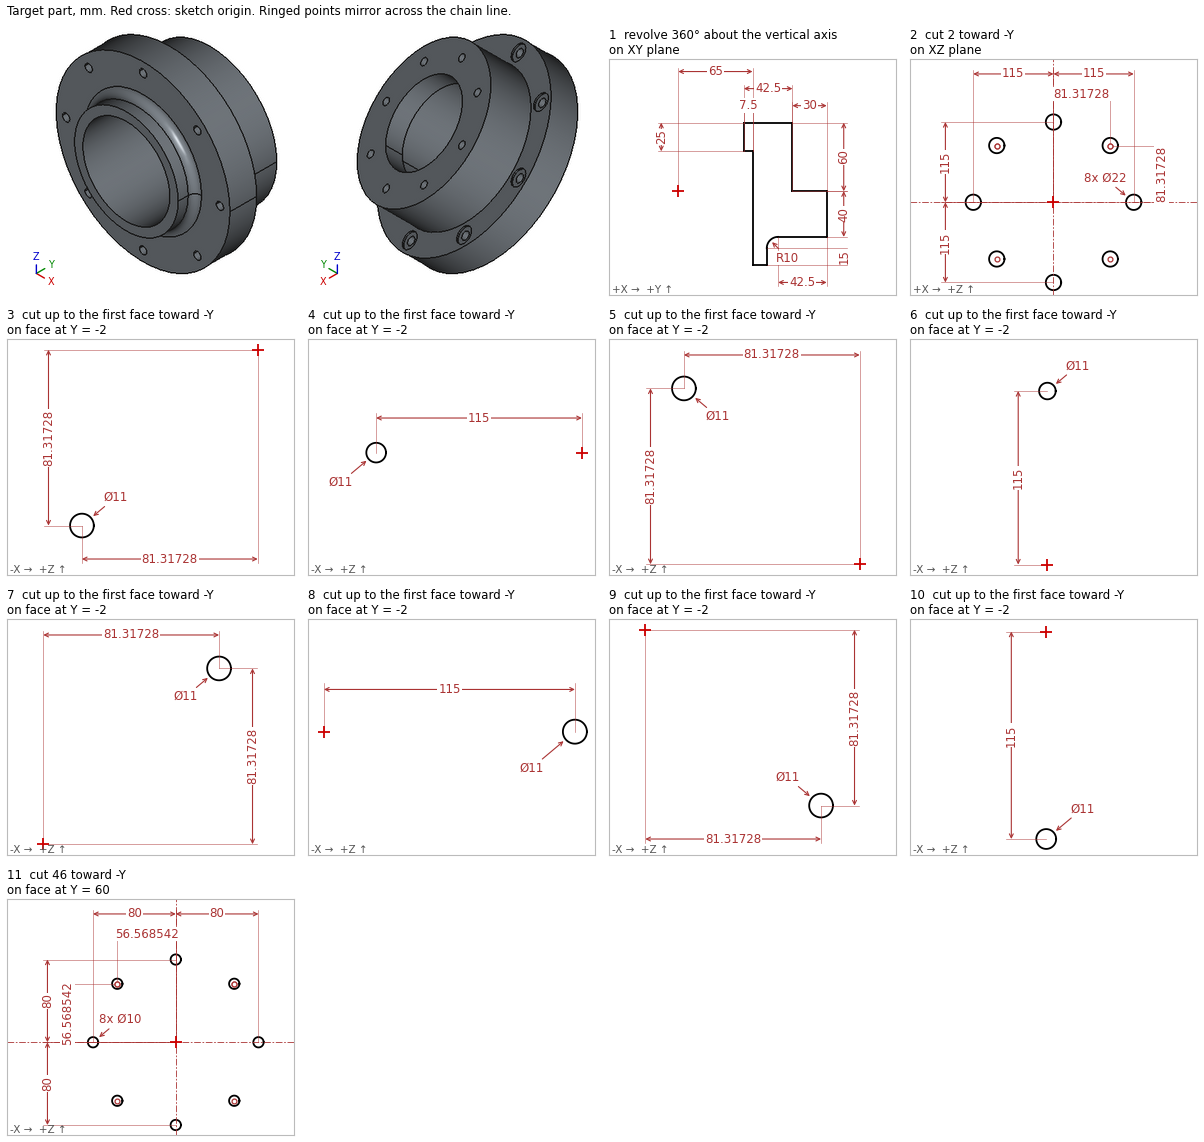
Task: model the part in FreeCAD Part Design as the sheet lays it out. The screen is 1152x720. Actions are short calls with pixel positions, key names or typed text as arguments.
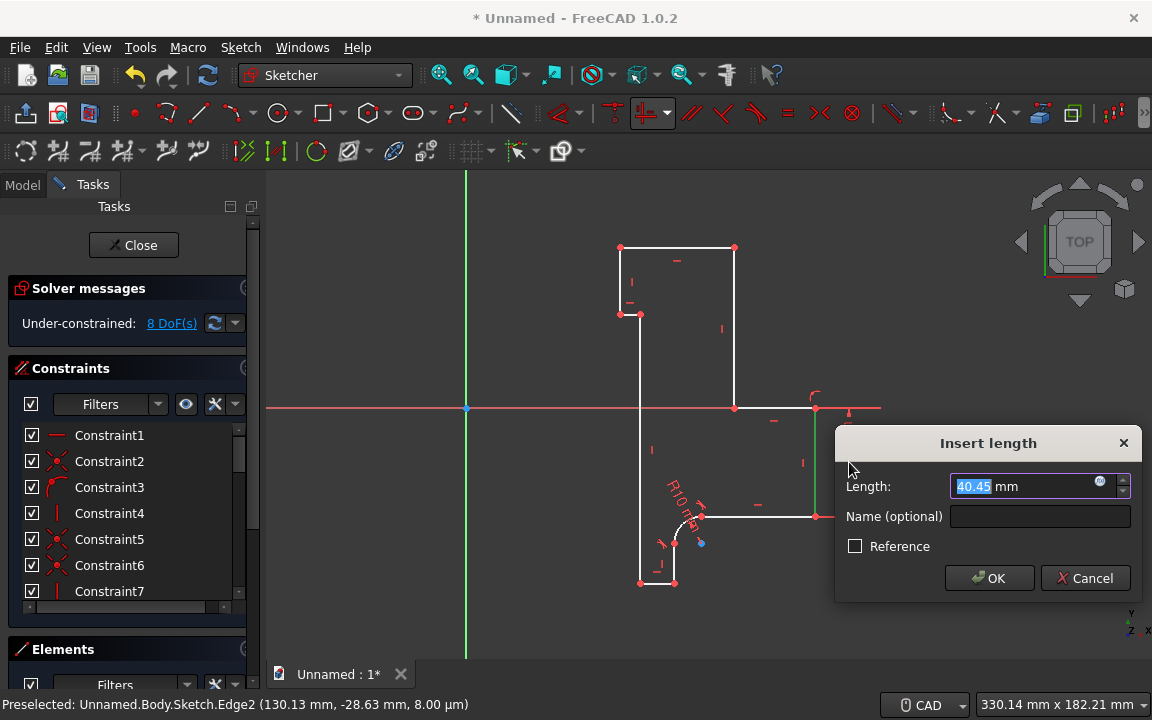
text(40)
key(Return)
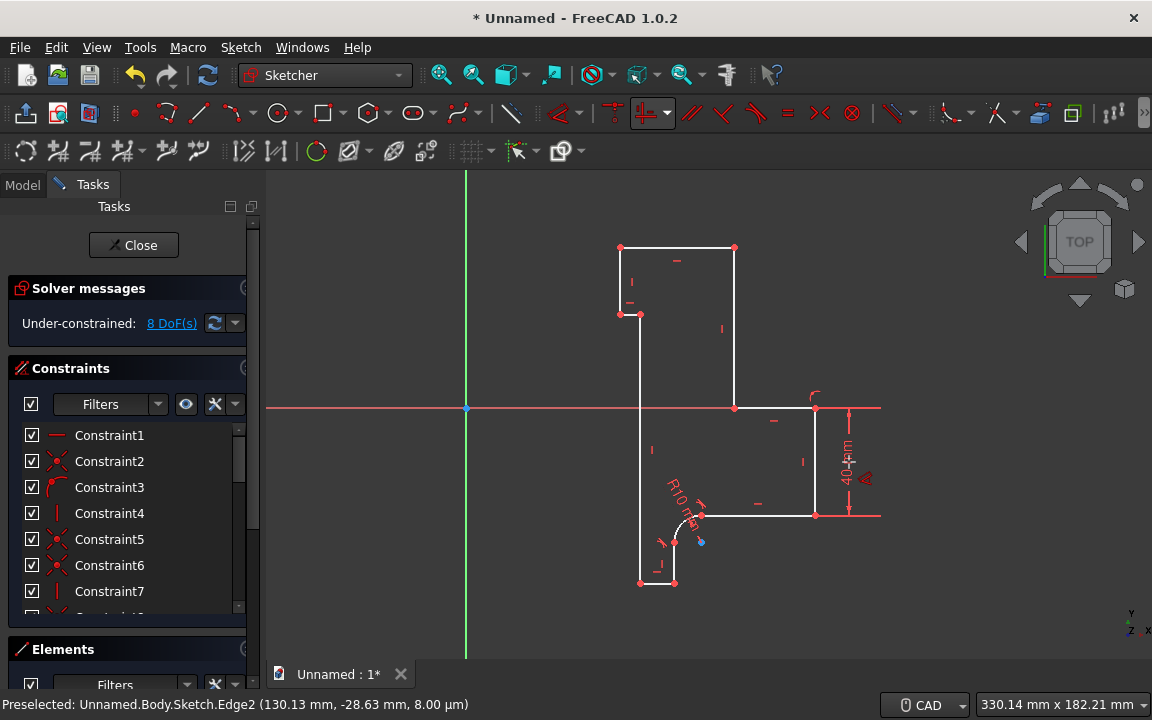
click(791, 408)
click(775, 374)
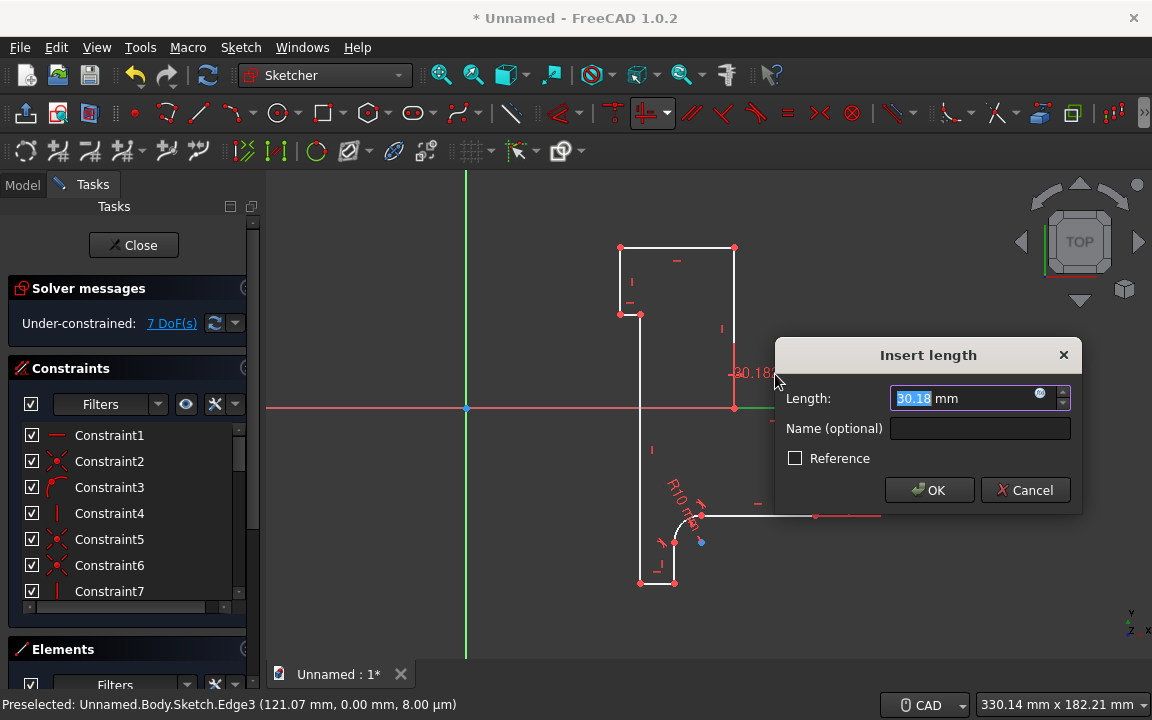
text(30)
key(Return)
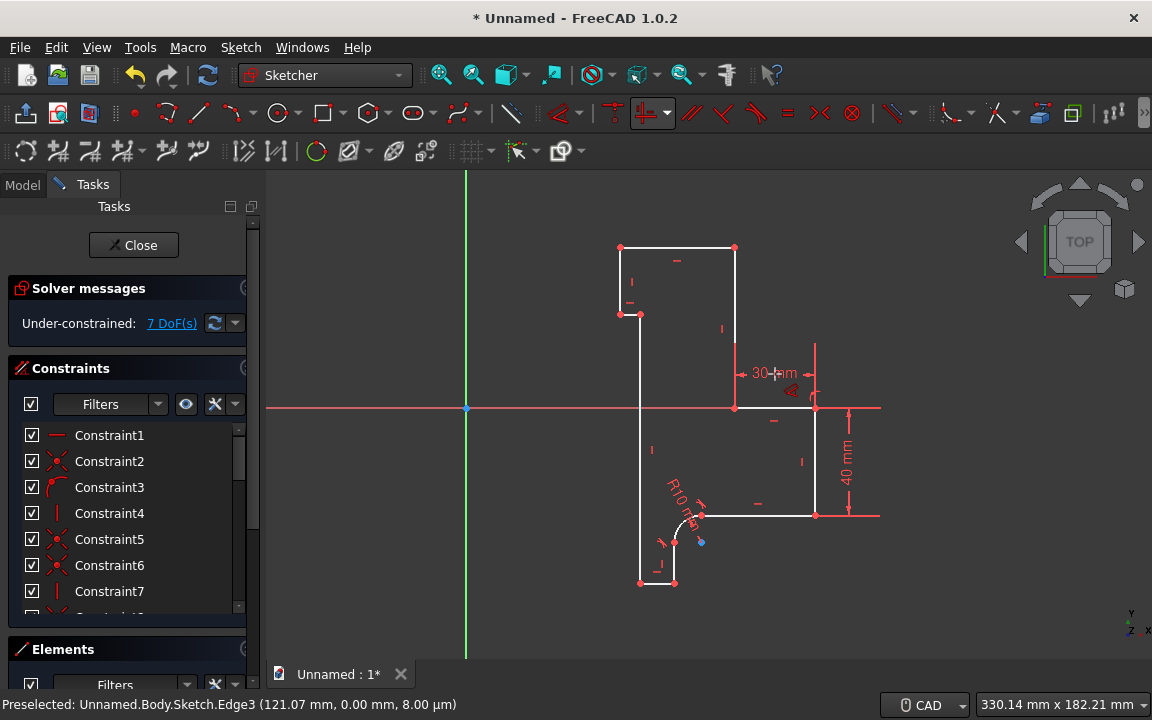
click(735, 360)
click(769, 328)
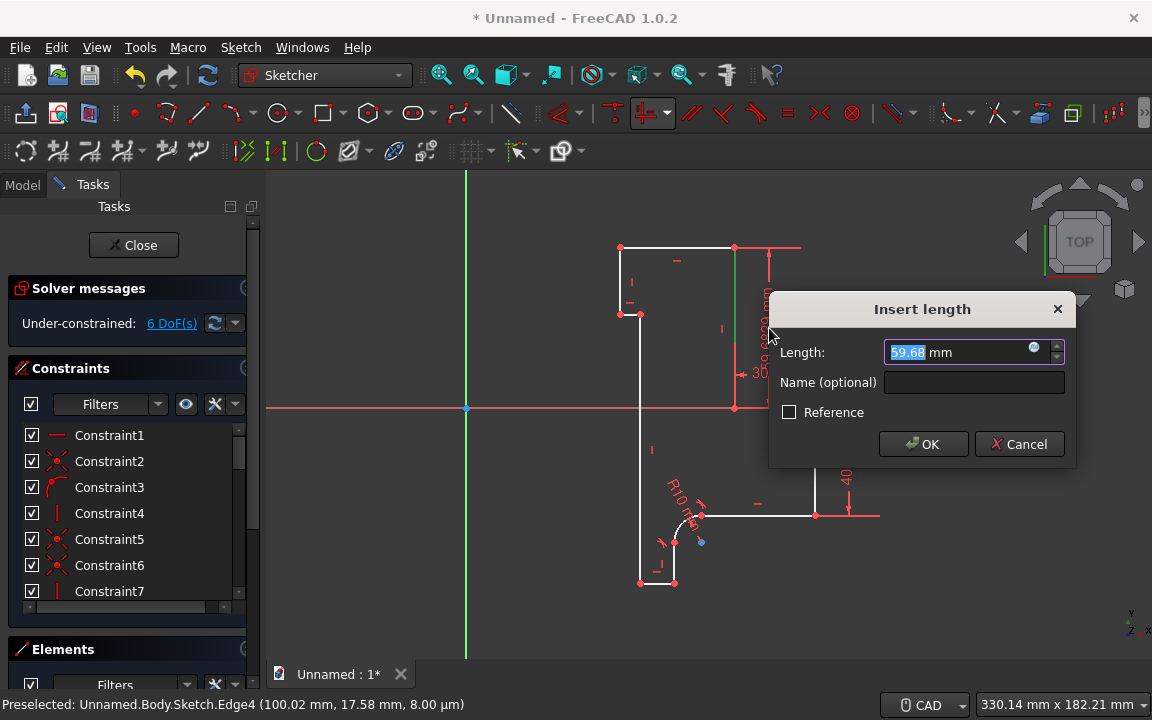
text(60)
key(Return)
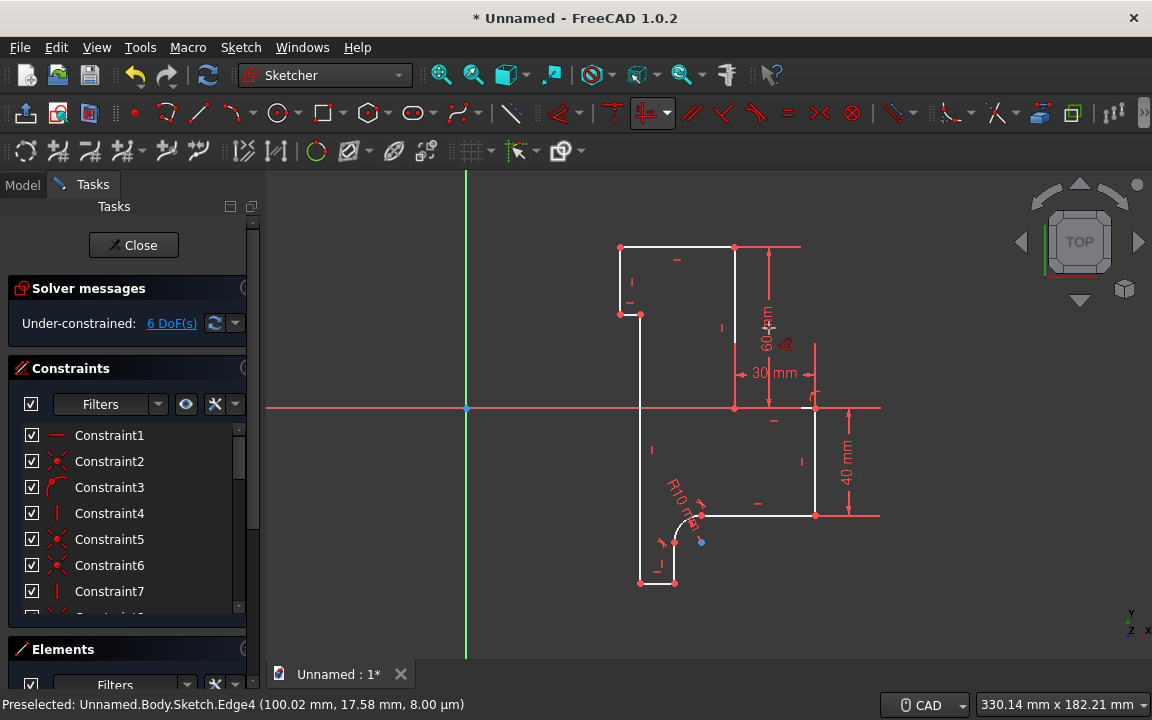
click(620, 268)
click(586, 281)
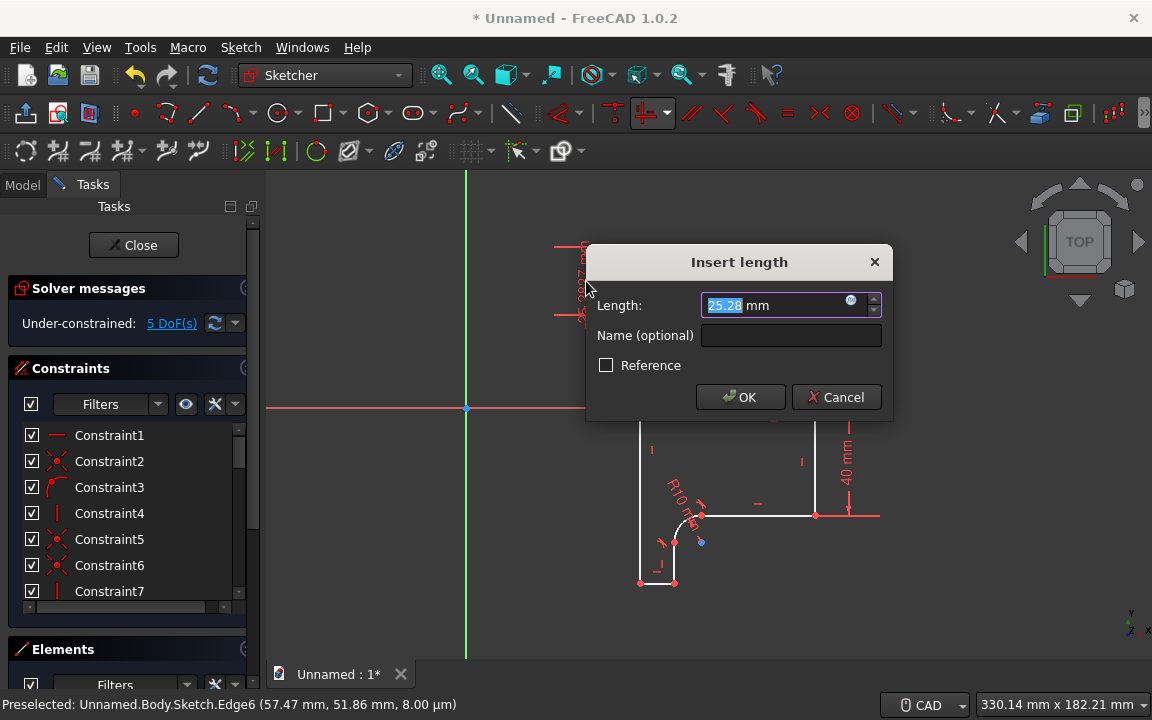
text(25)
key(Return)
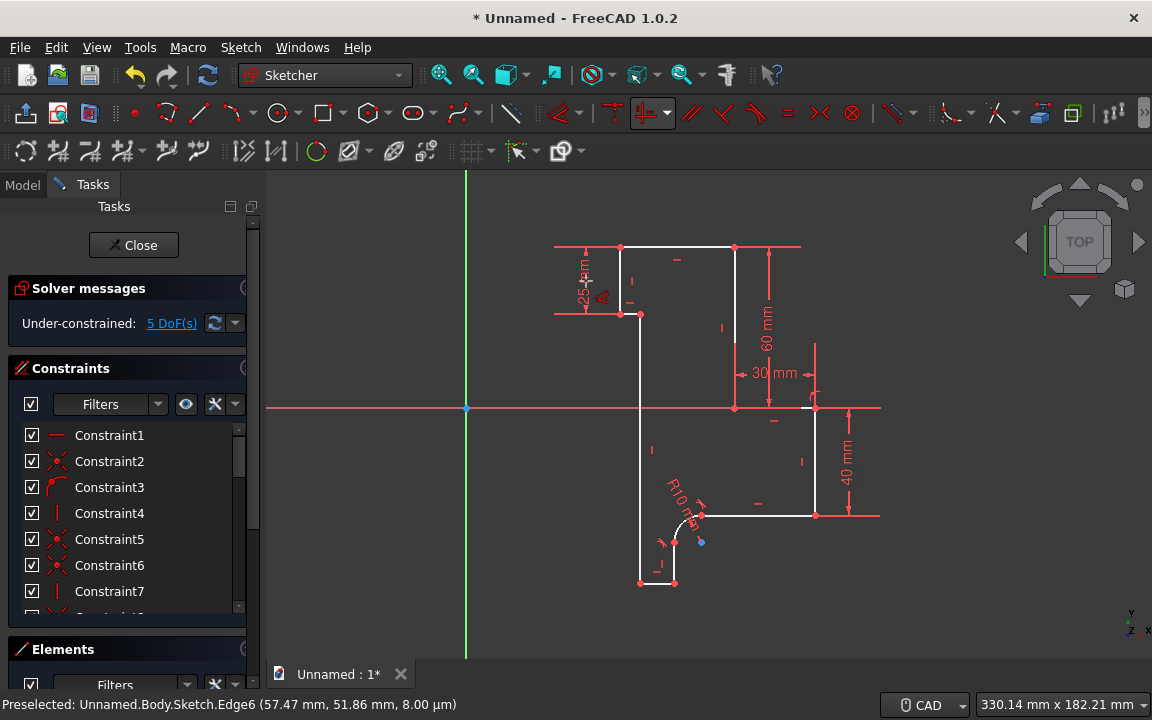
click(674, 572)
click(708, 563)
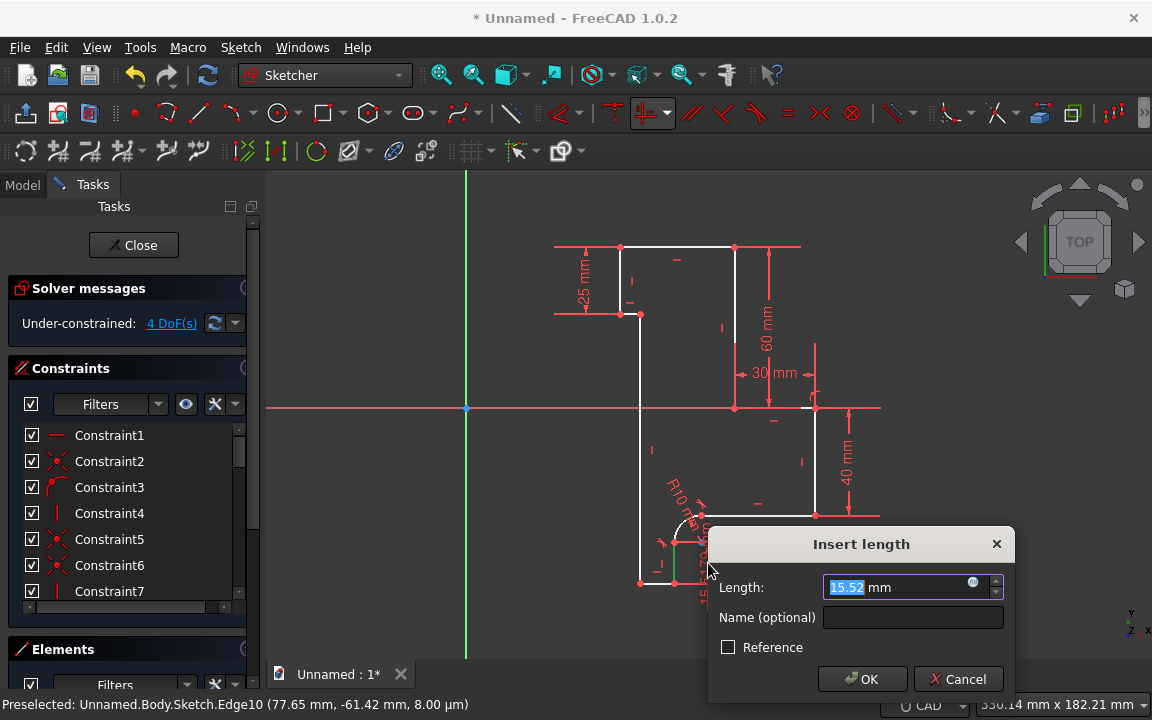
text(15)
key(Return)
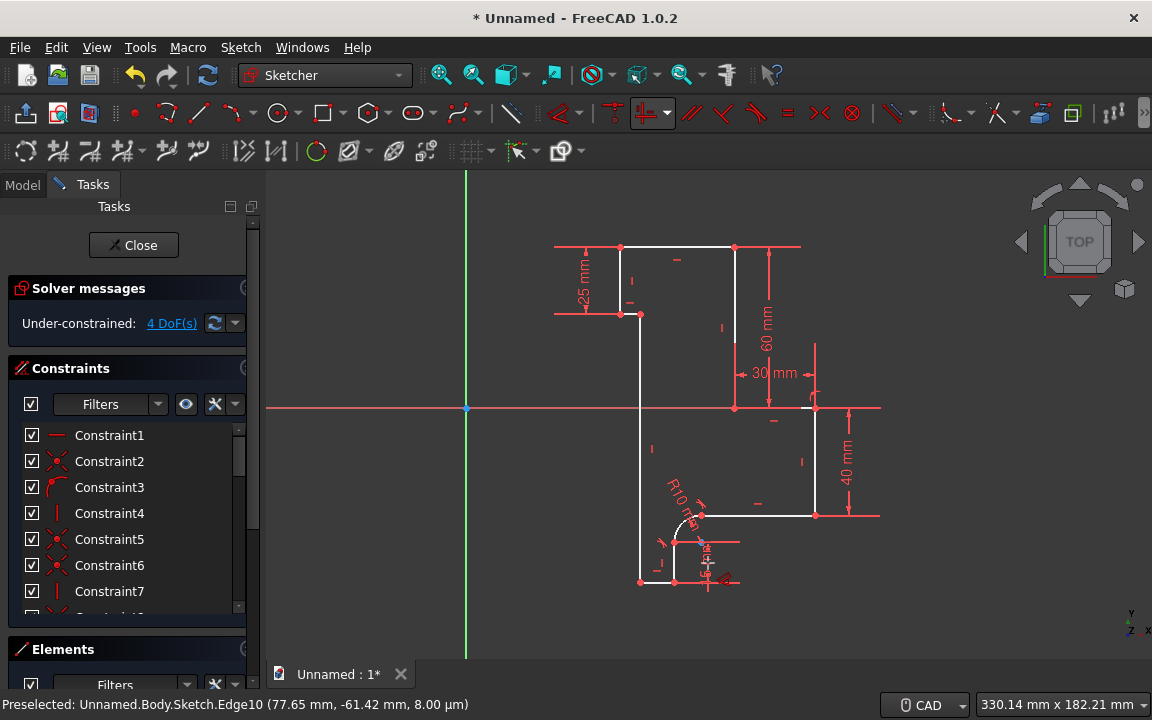
scroll(630, 314, up, 4)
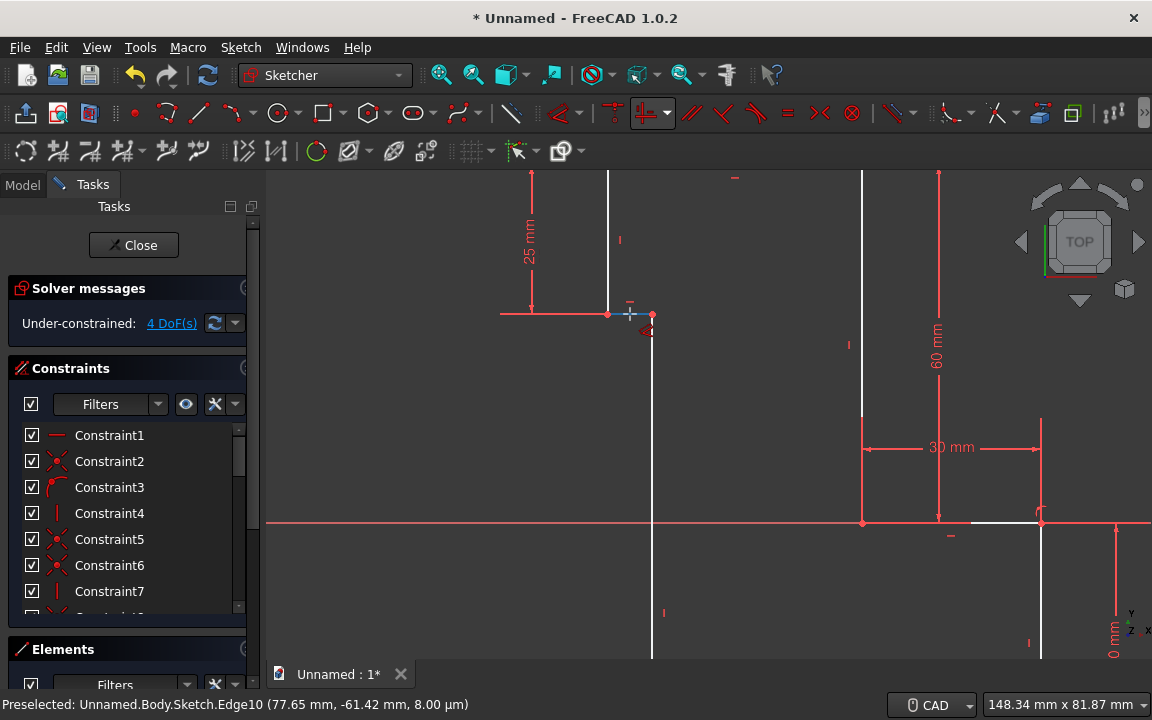
click(630, 314)
click(630, 280)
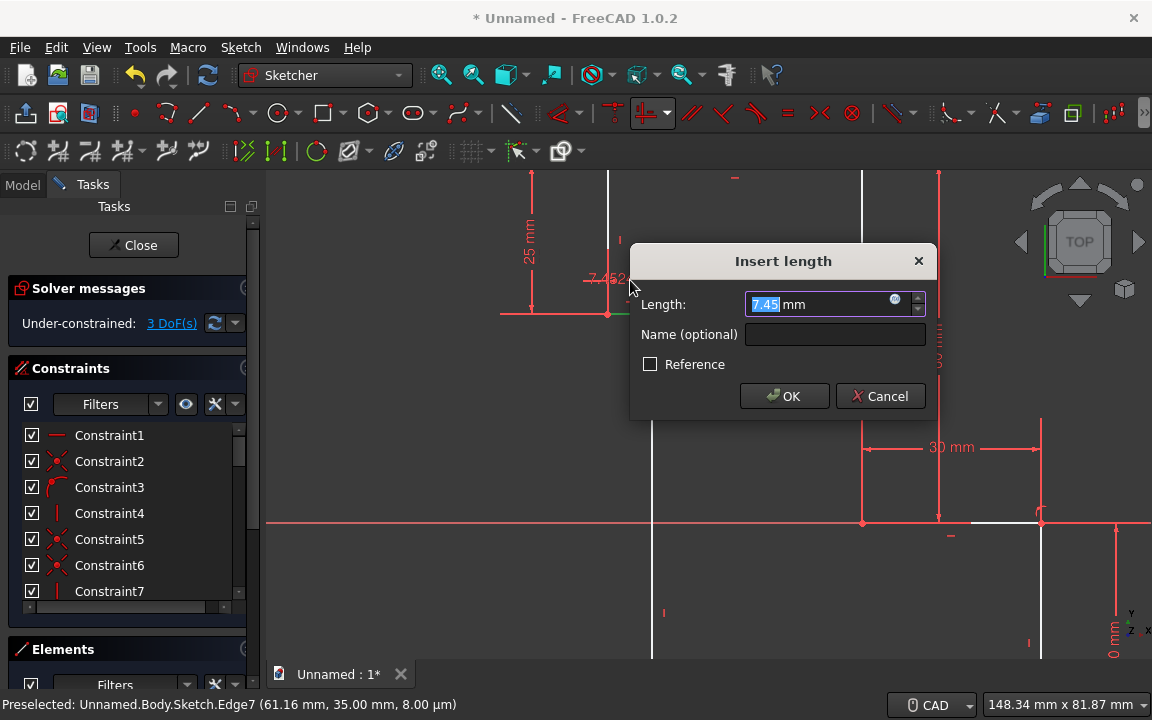
text(7.5)
key(Return)